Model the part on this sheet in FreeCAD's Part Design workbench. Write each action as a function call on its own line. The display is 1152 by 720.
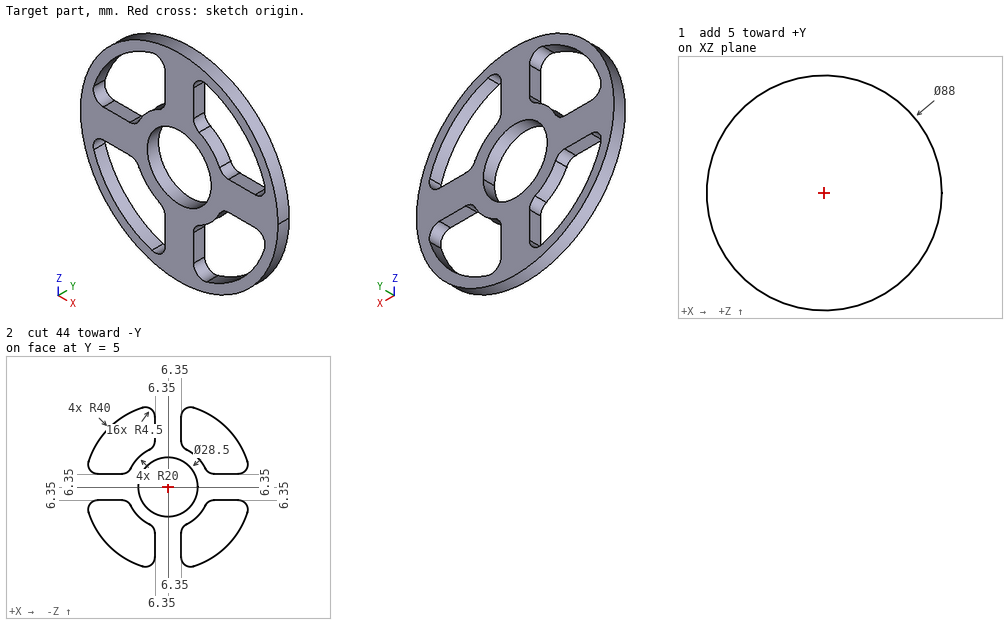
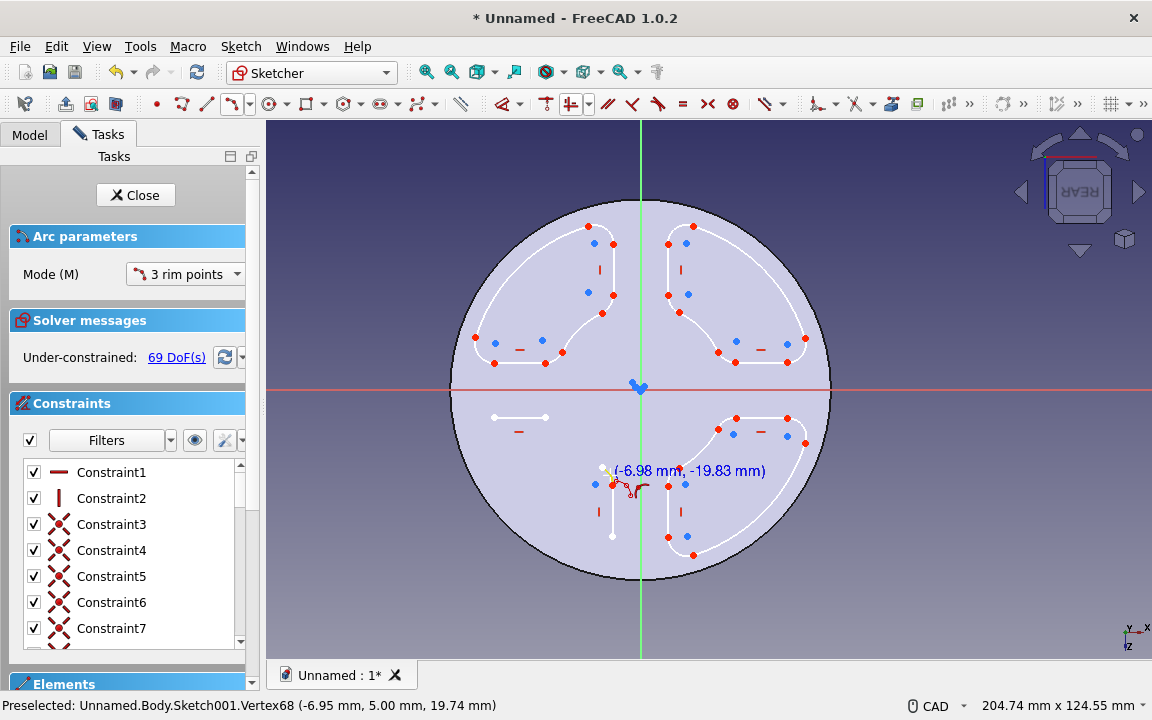
click(602, 468)
click(563, 428)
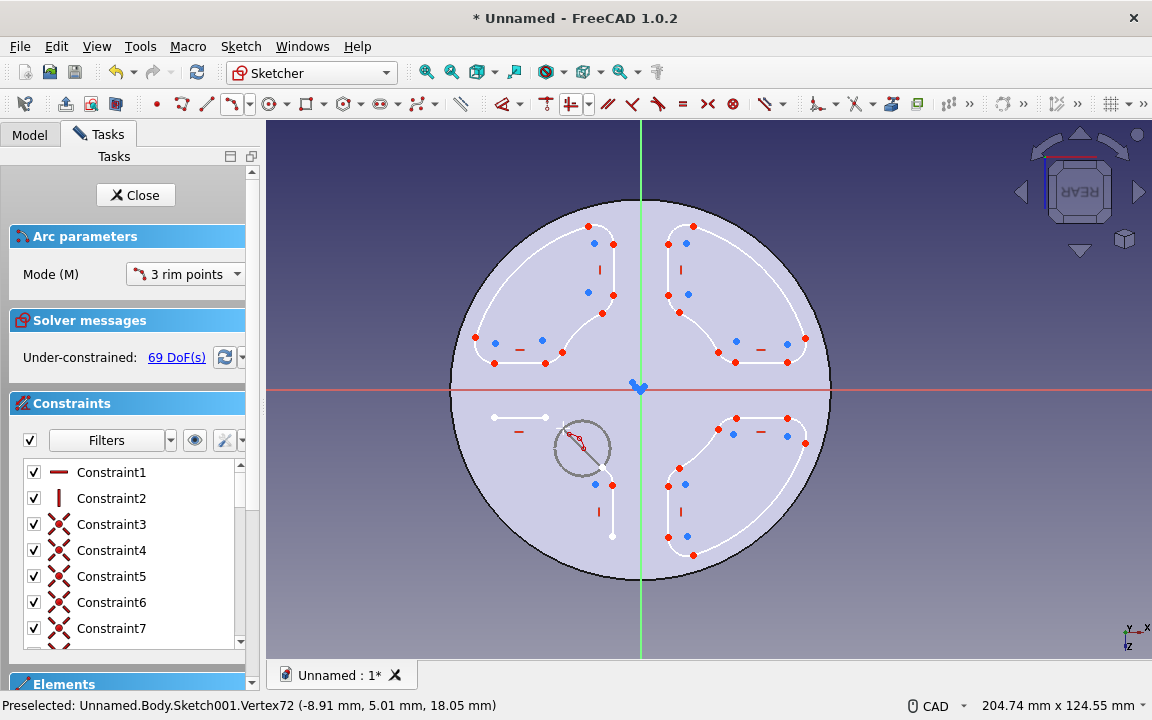
scroll(579, 451, up, 7)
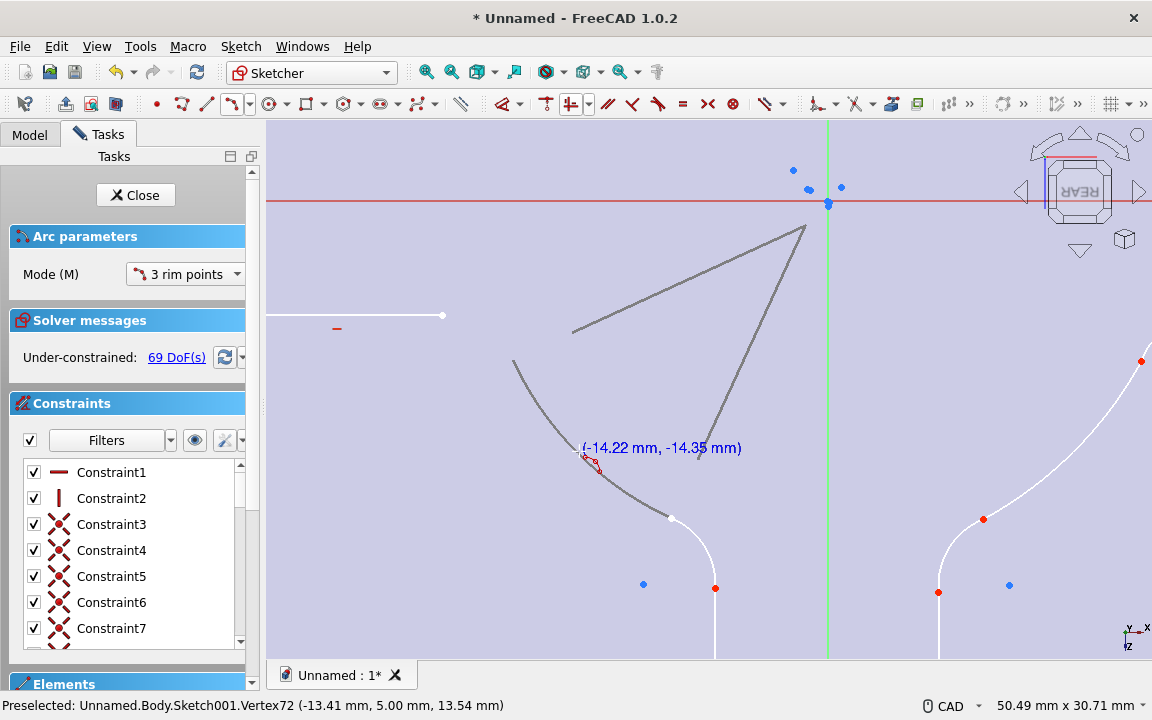
click(579, 450)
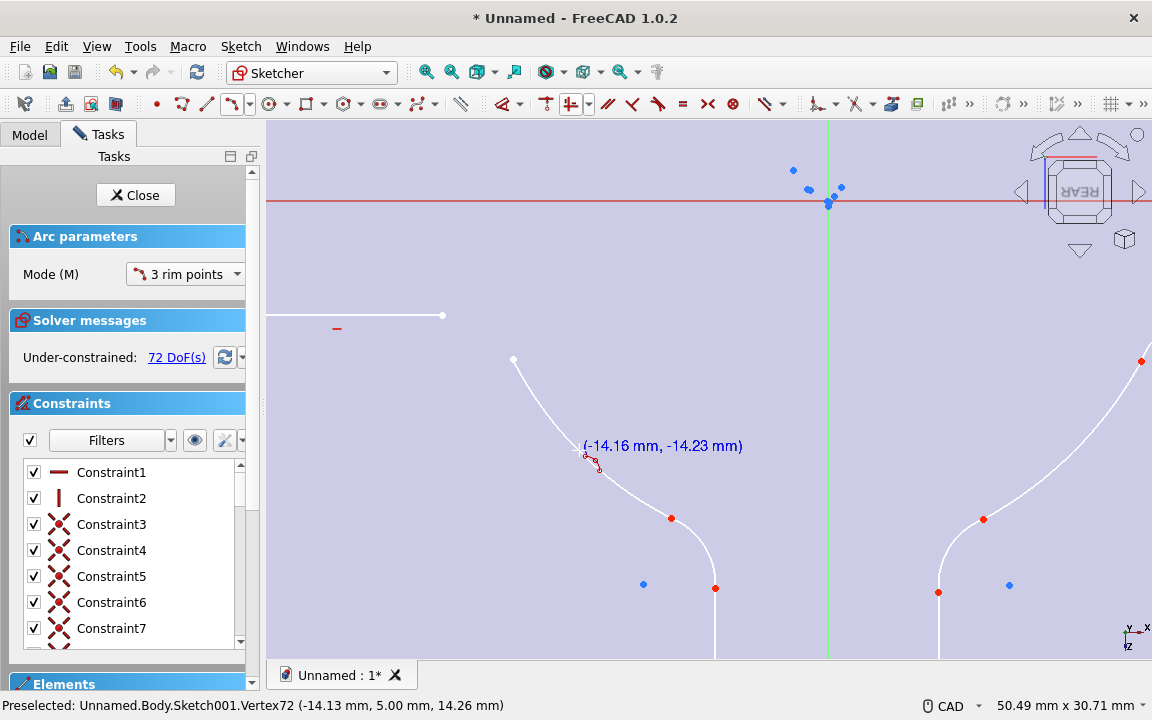
scroll(579, 451, down, 7)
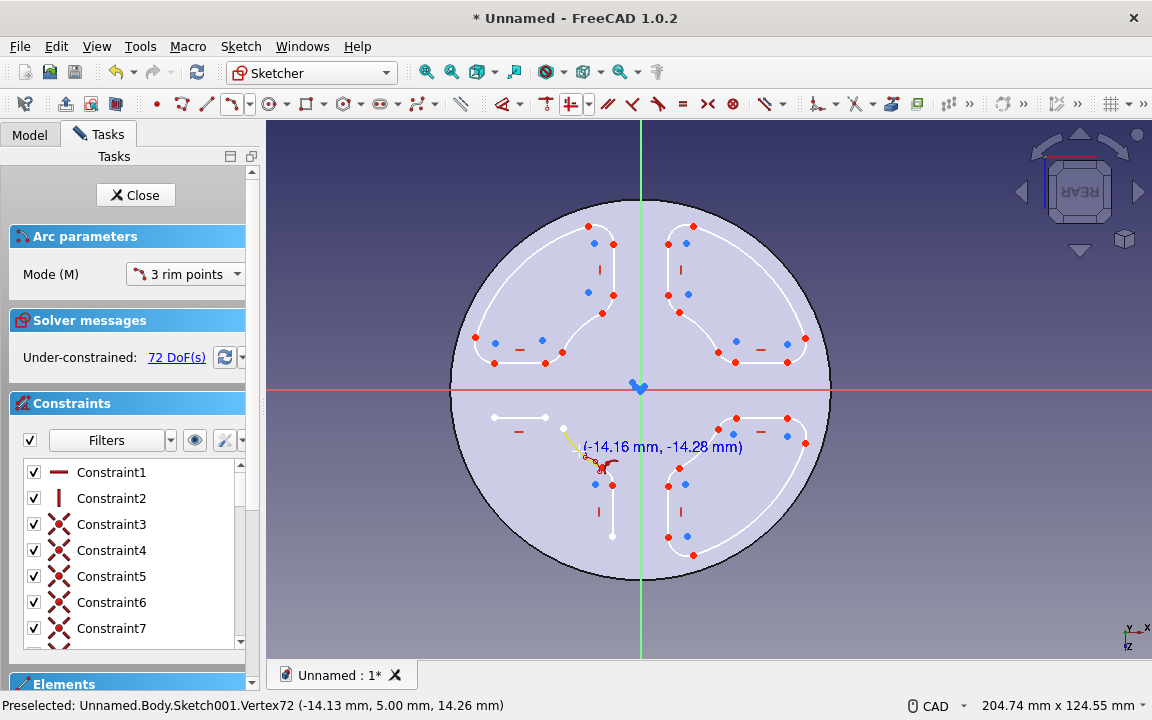
click(563, 429)
click(546, 418)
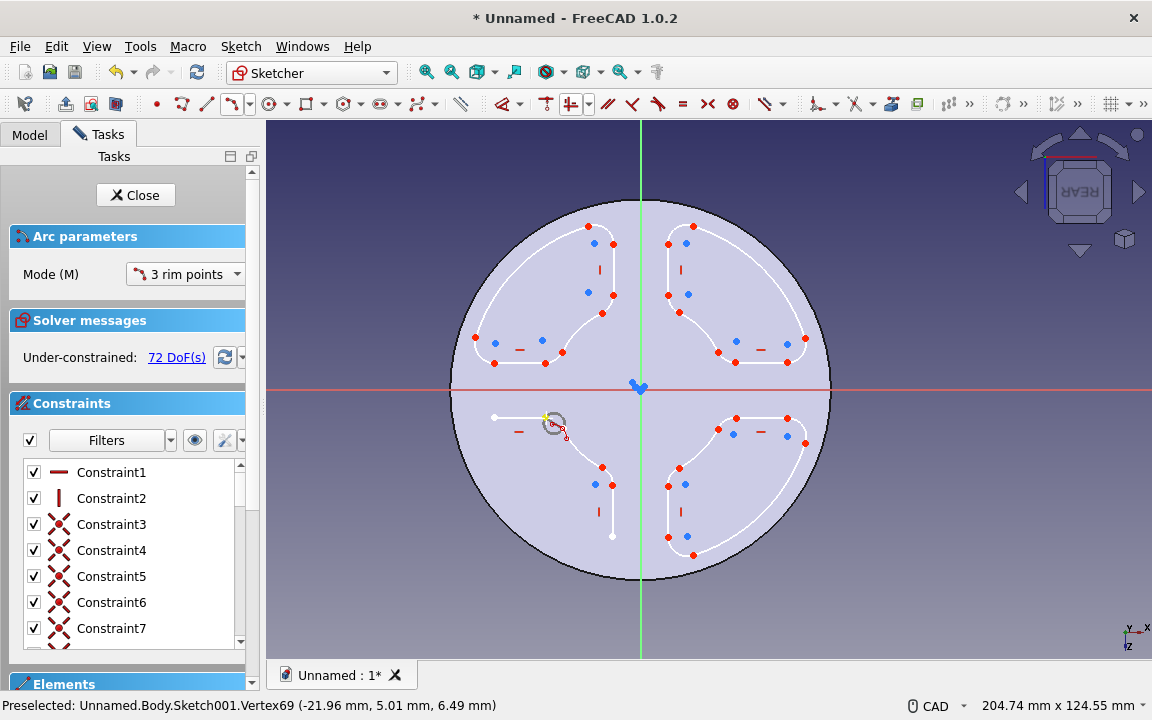
scroll(556, 420, up, 9)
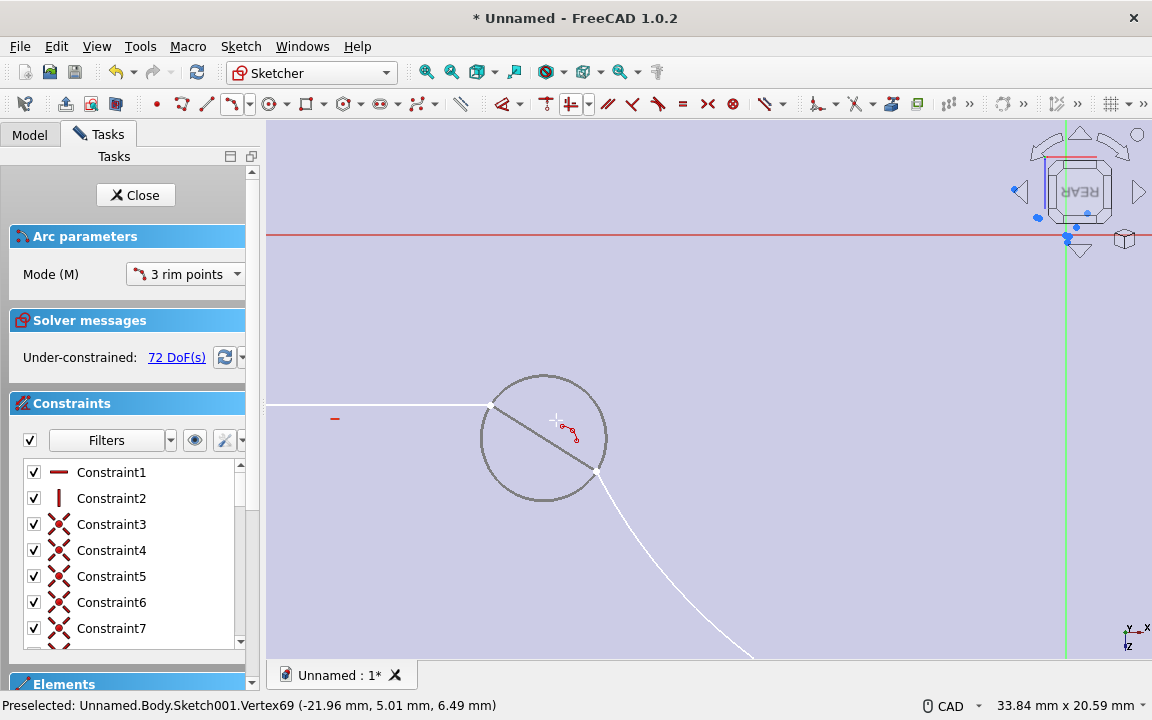
click(553, 419)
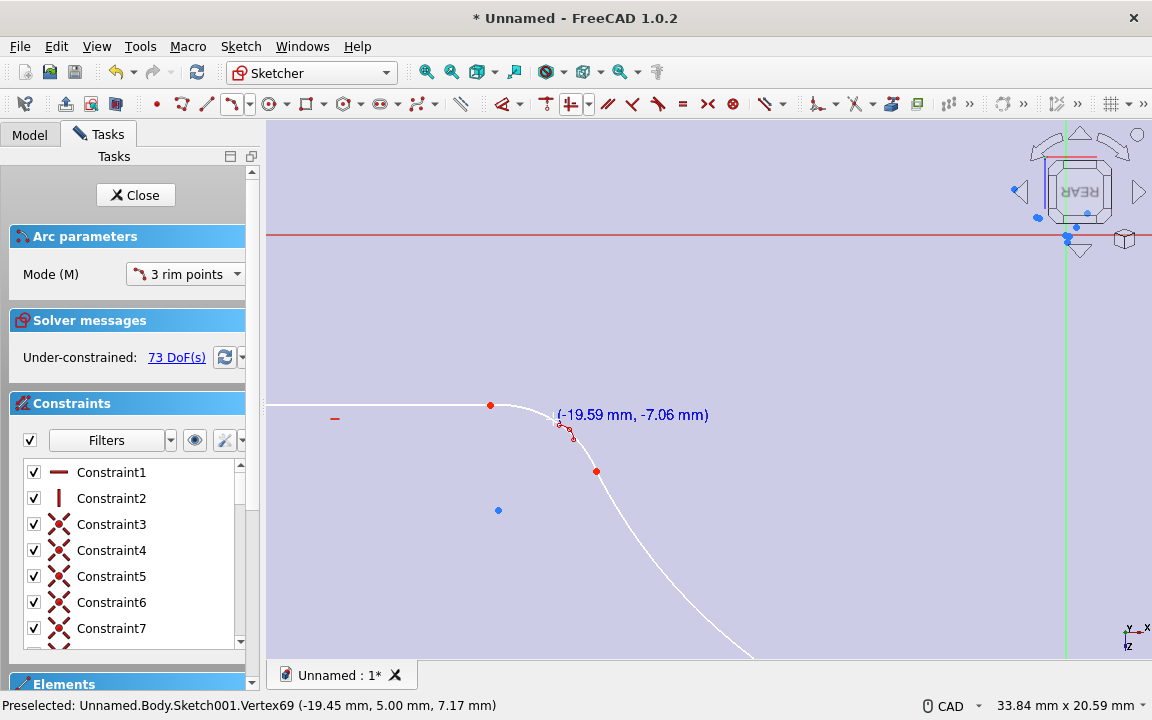
scroll(556, 420, down, 9)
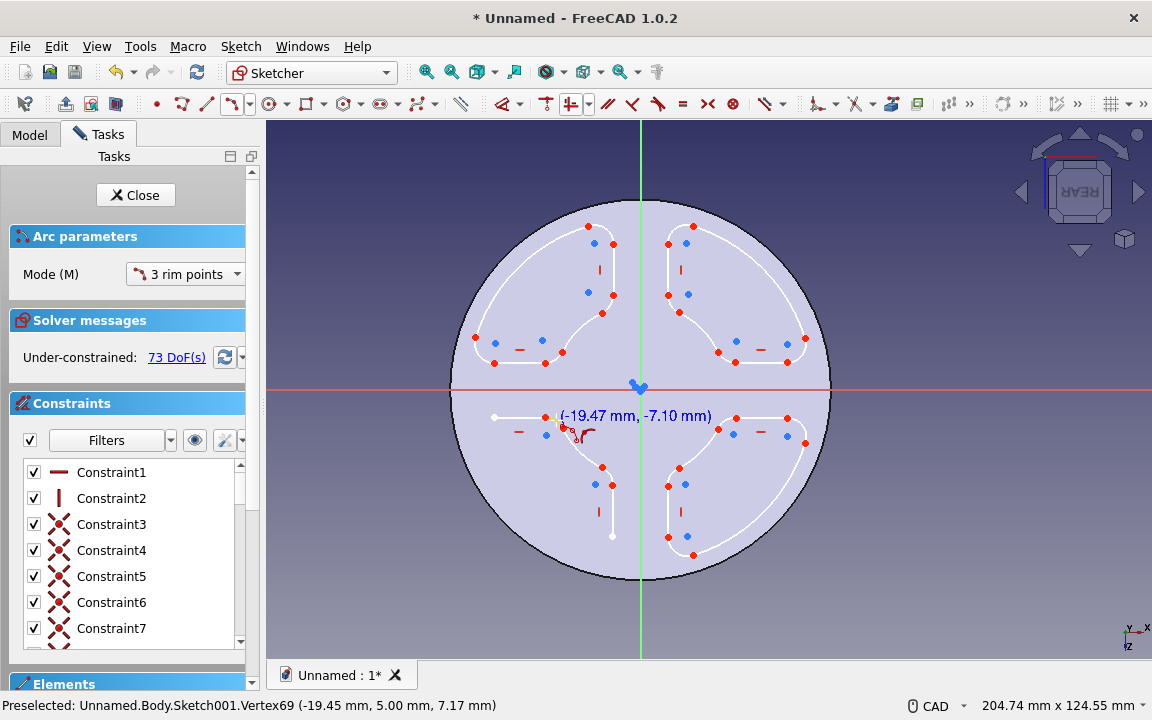
click(494, 418)
click(476, 443)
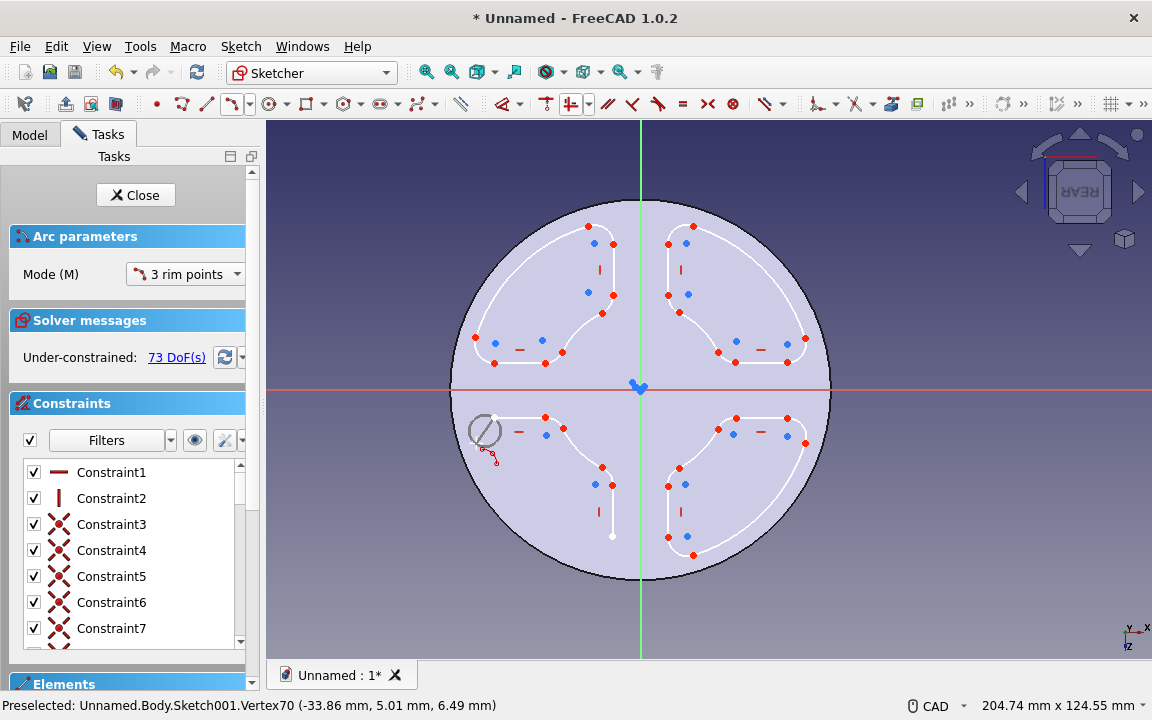
scroll(479, 425, up, 4)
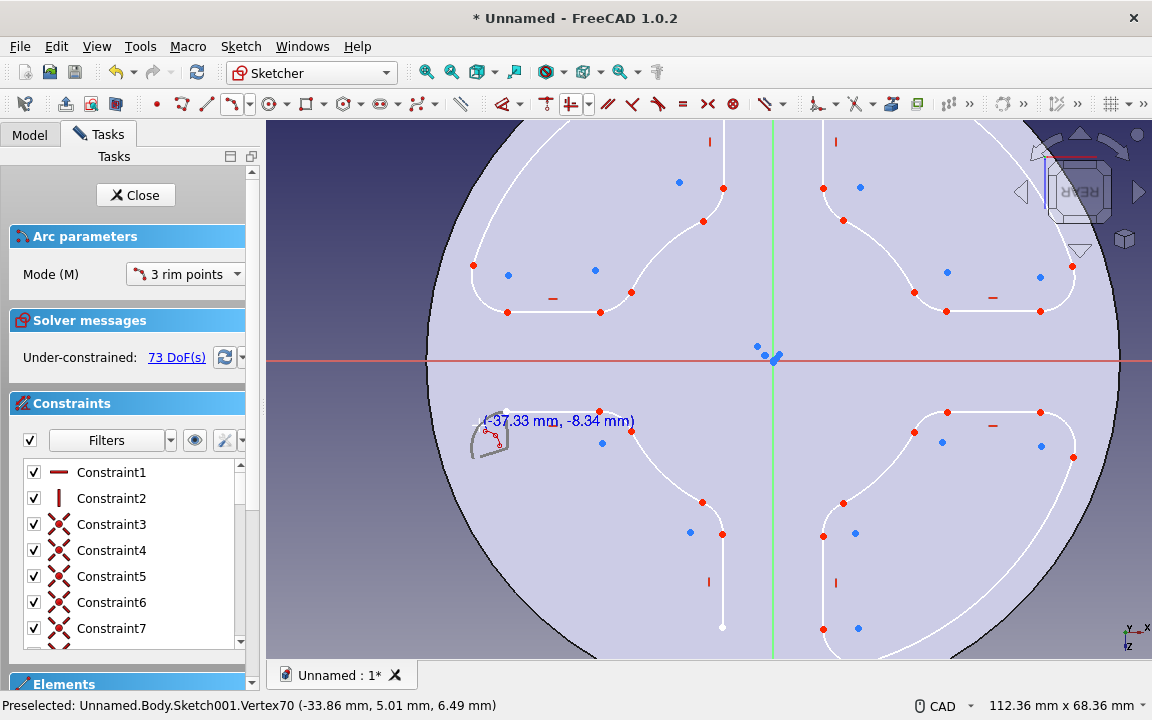
click(478, 425)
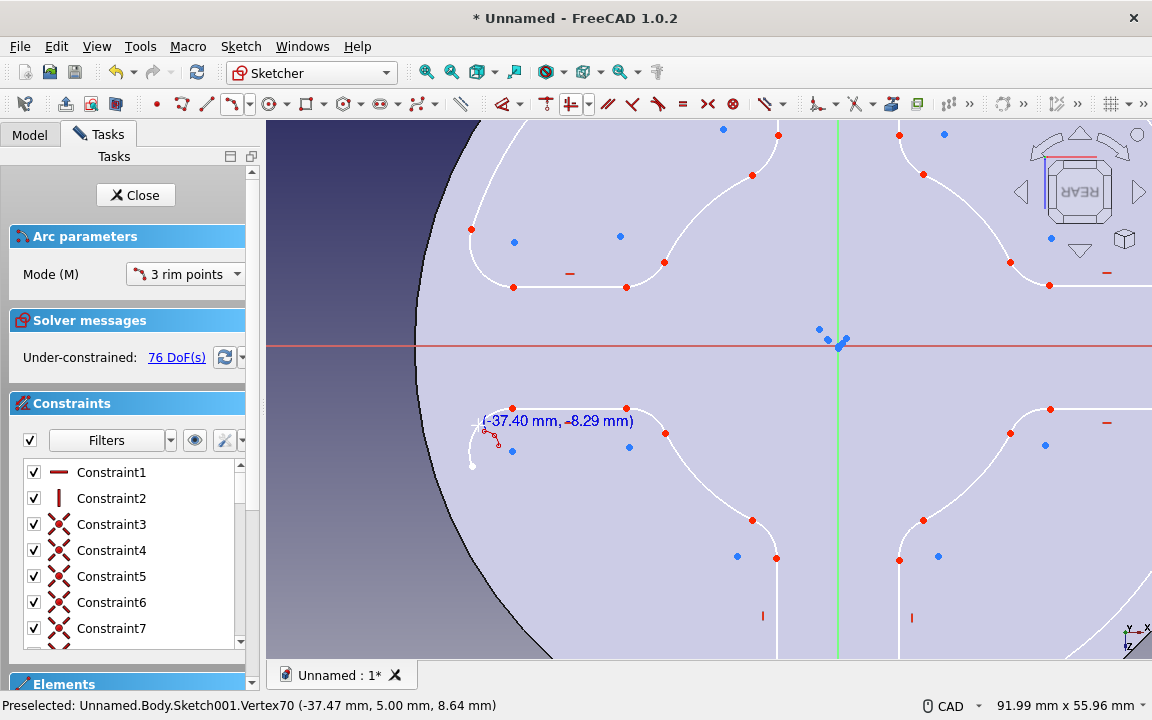
click(472, 467)